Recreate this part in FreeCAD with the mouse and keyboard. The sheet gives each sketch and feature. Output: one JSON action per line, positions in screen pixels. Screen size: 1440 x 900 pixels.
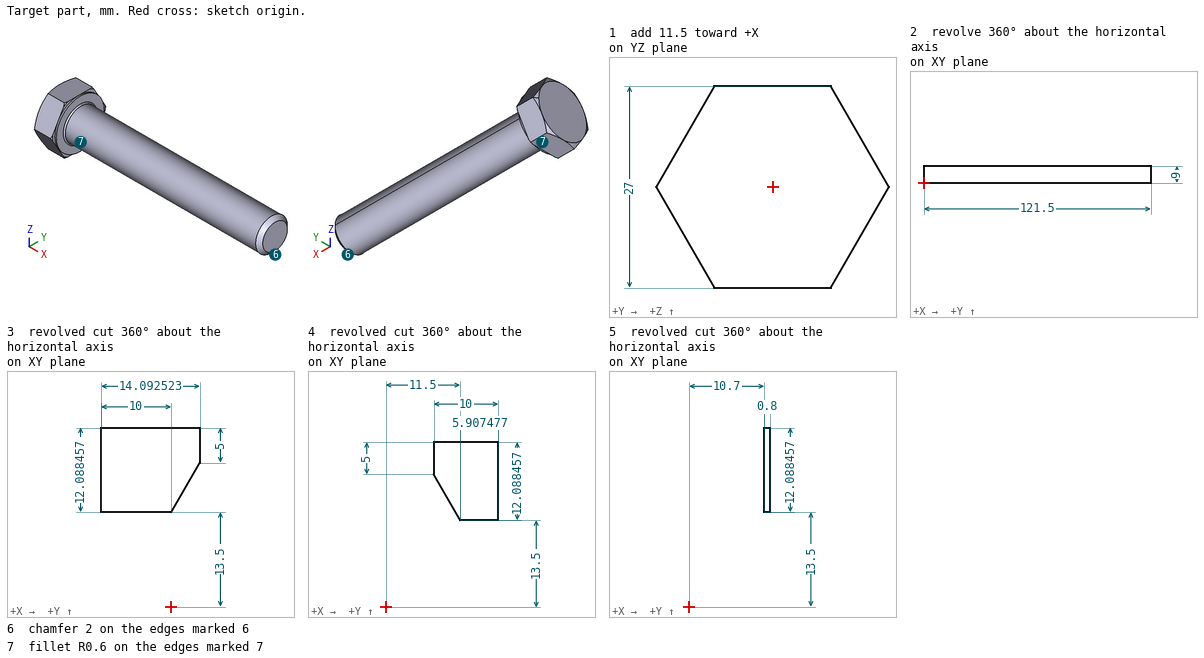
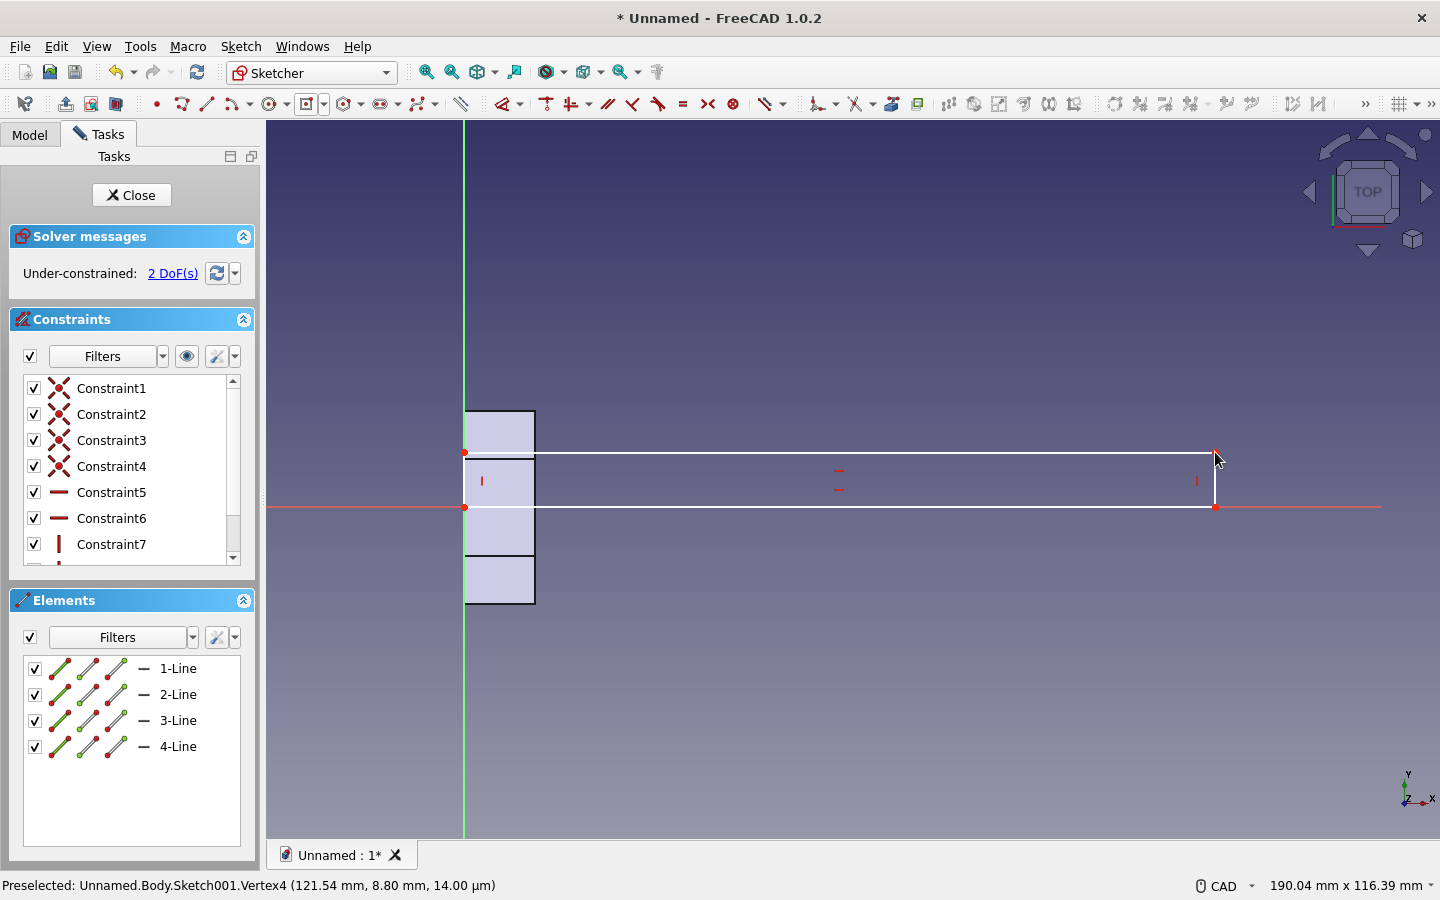
{"action": "left_click", "coordinate": [502, 104]}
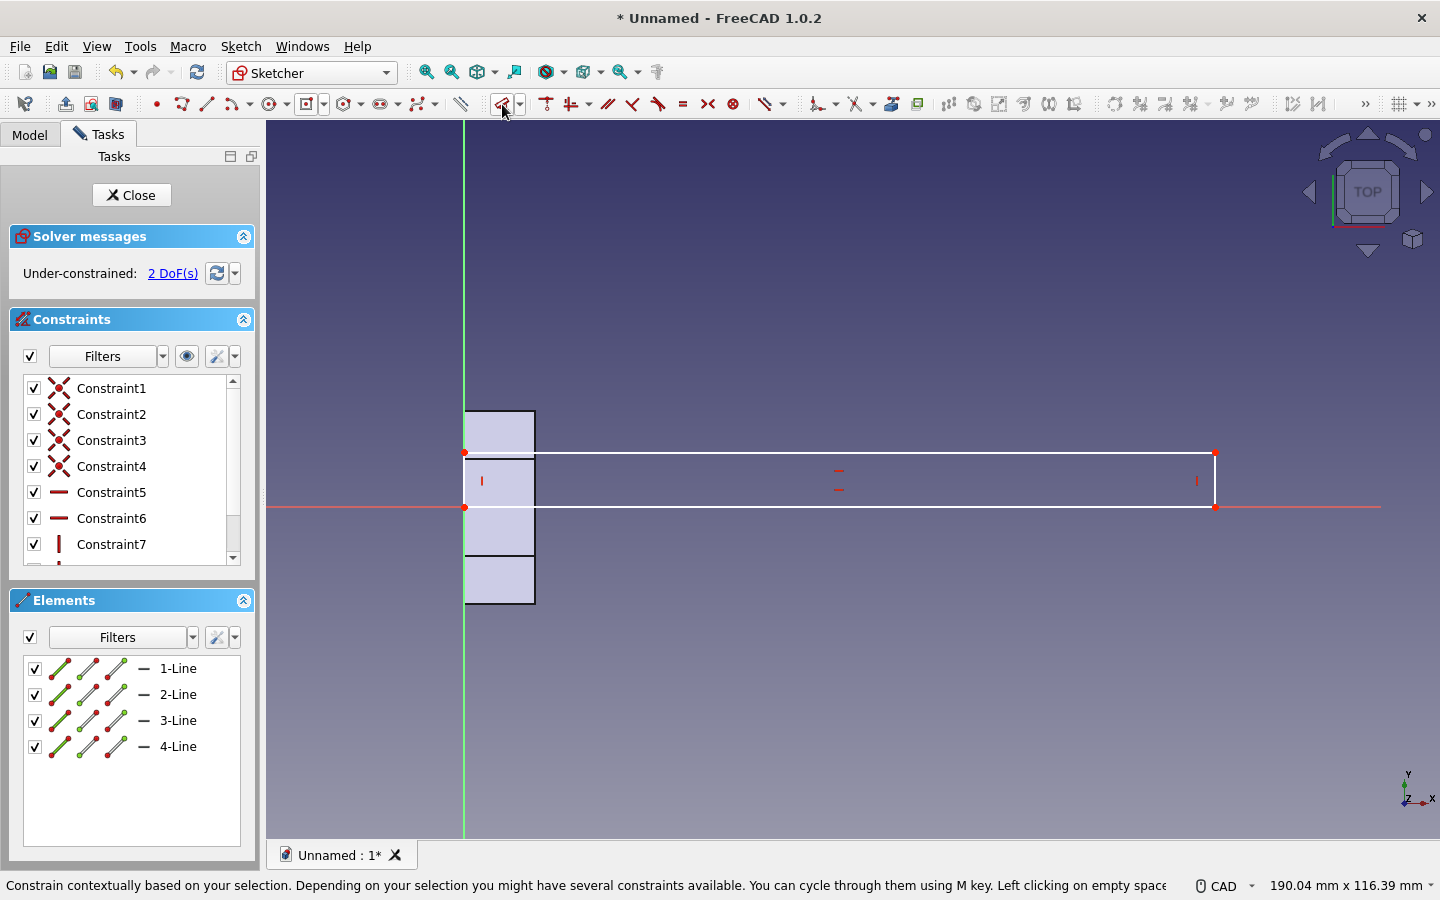
{"action": "left_click", "coordinate": [1215, 491]}
{"action": "left_click", "coordinate": [1249, 480]}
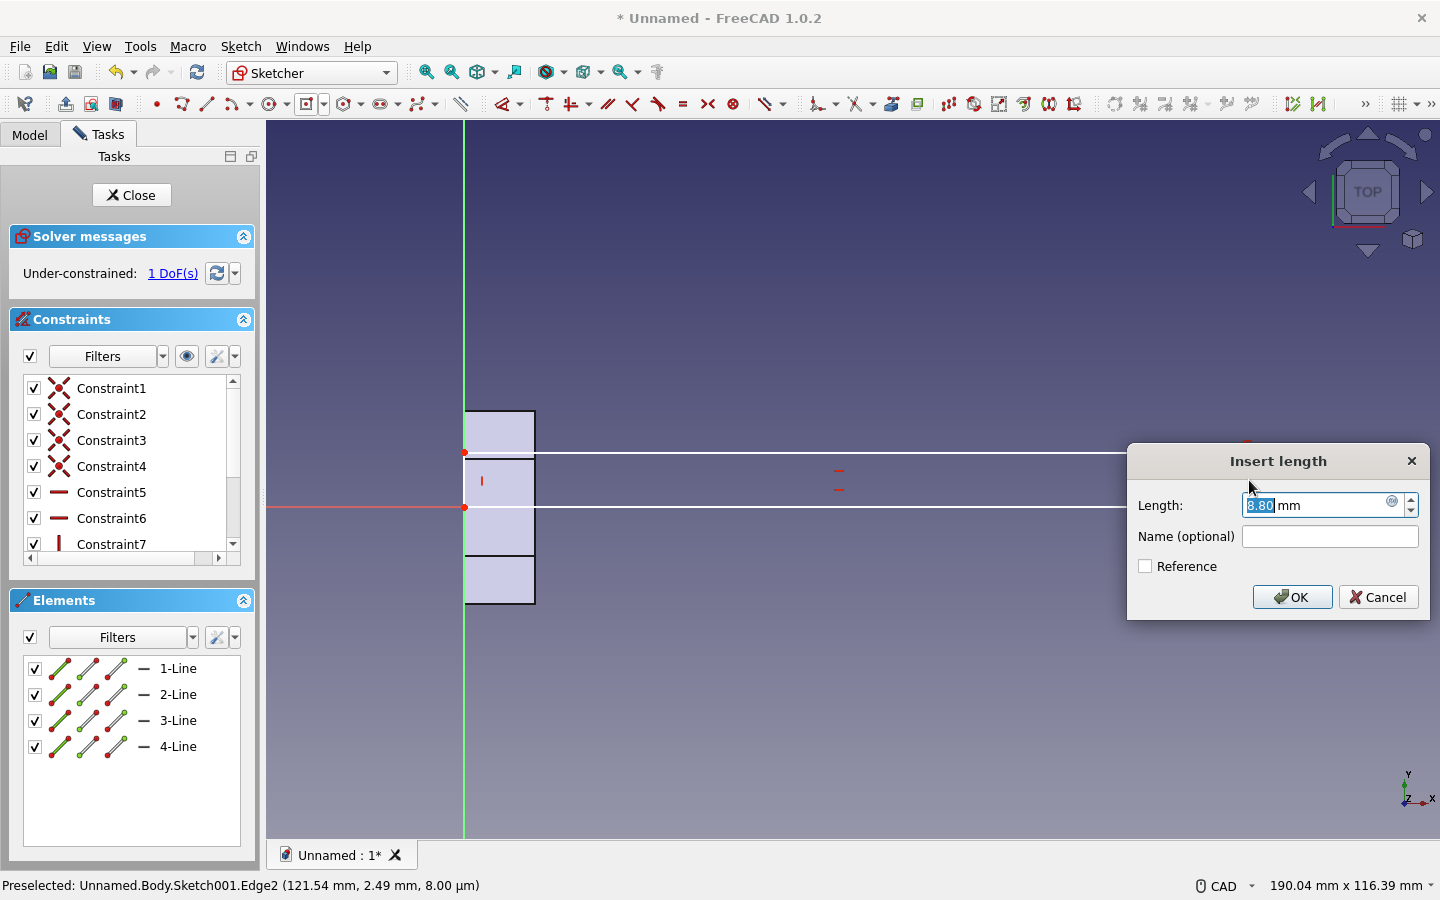
{"action": "type", "text": "9"}
{"action": "key", "text": "Return"}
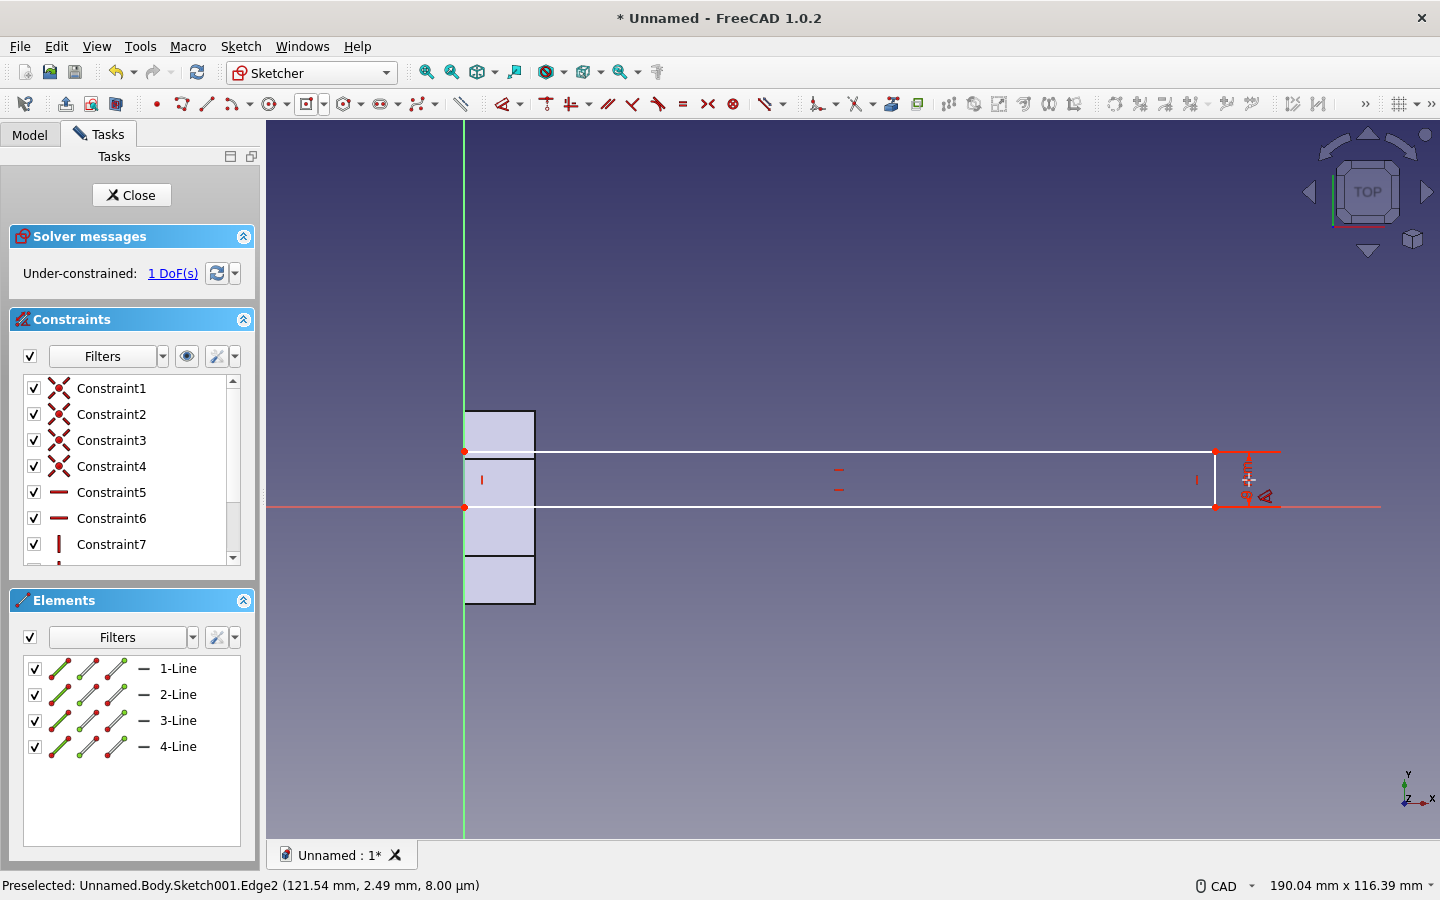
{"action": "left_click", "coordinate": [689, 507]}
{"action": "left_click", "coordinate": [840, 541]}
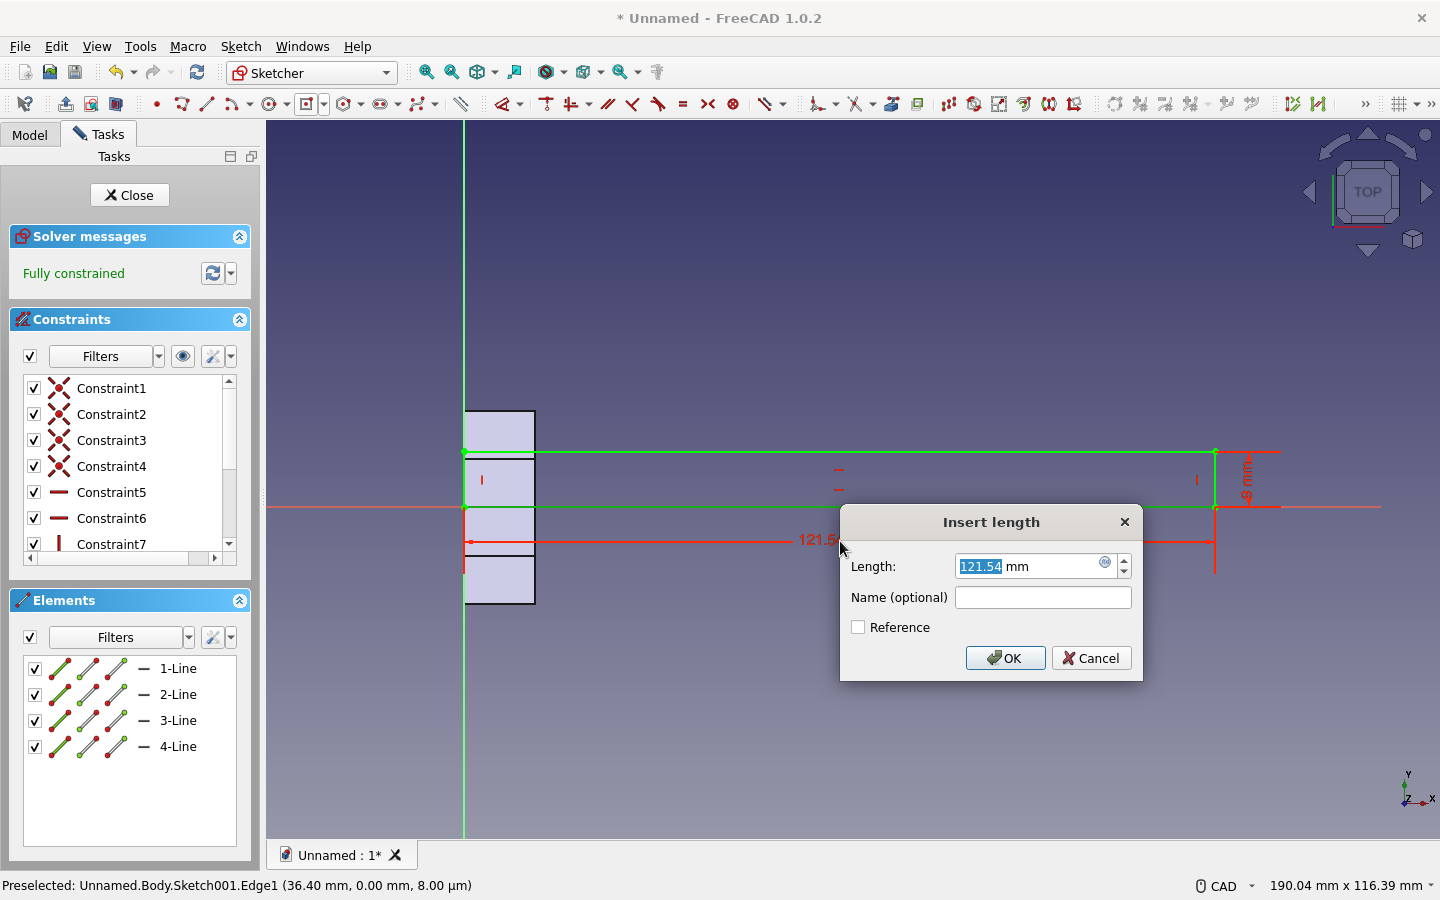
{"action": "type", "text": "121.5"}
{"action": "key", "text": "Return"}
{"action": "key", "text": "Escape"}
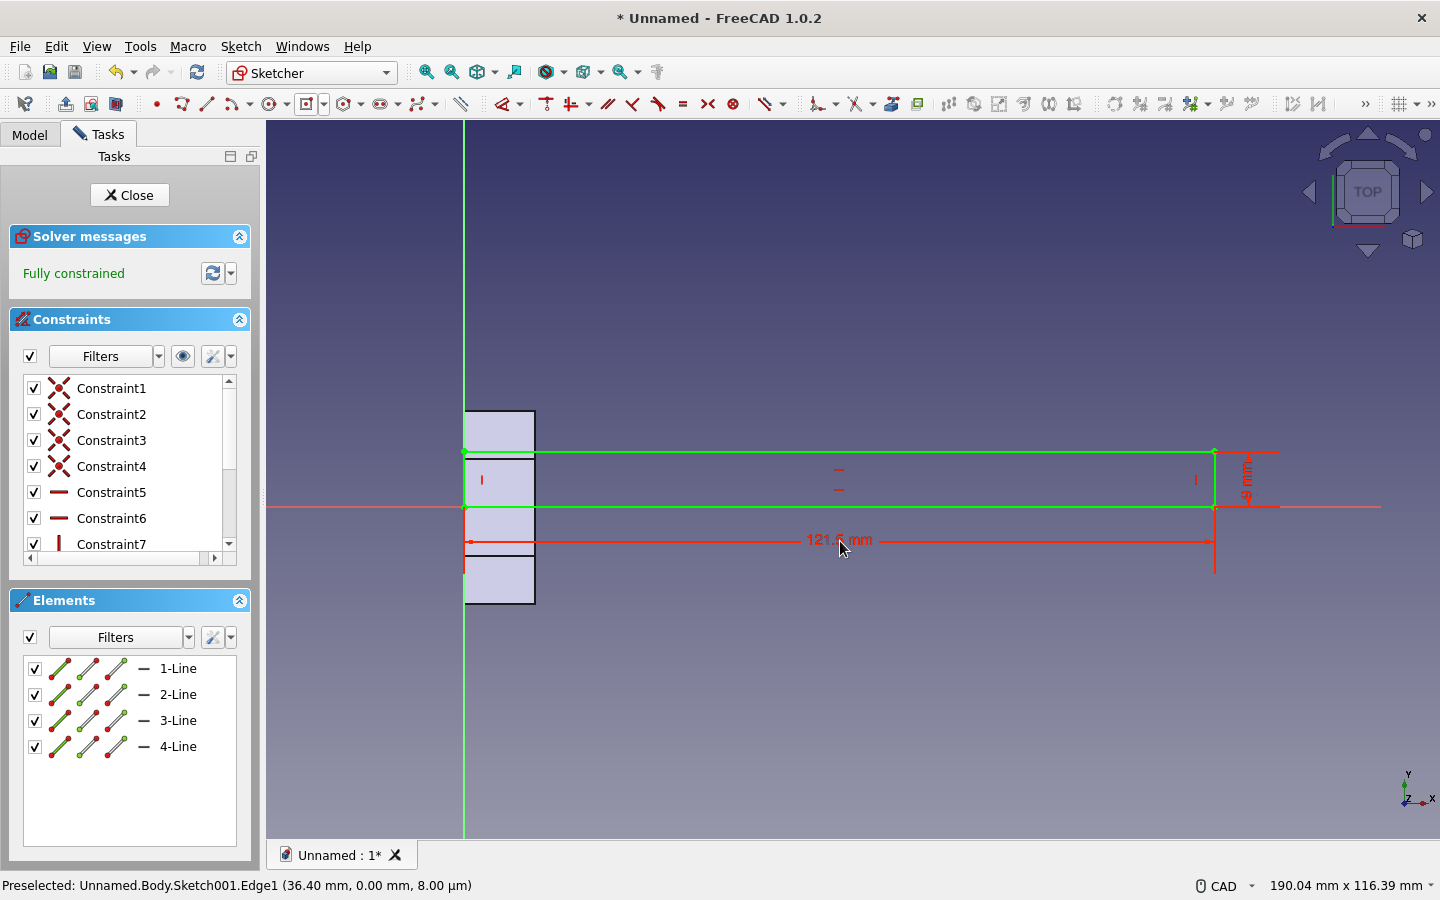
{"action": "left_click", "coordinate": [130, 195]}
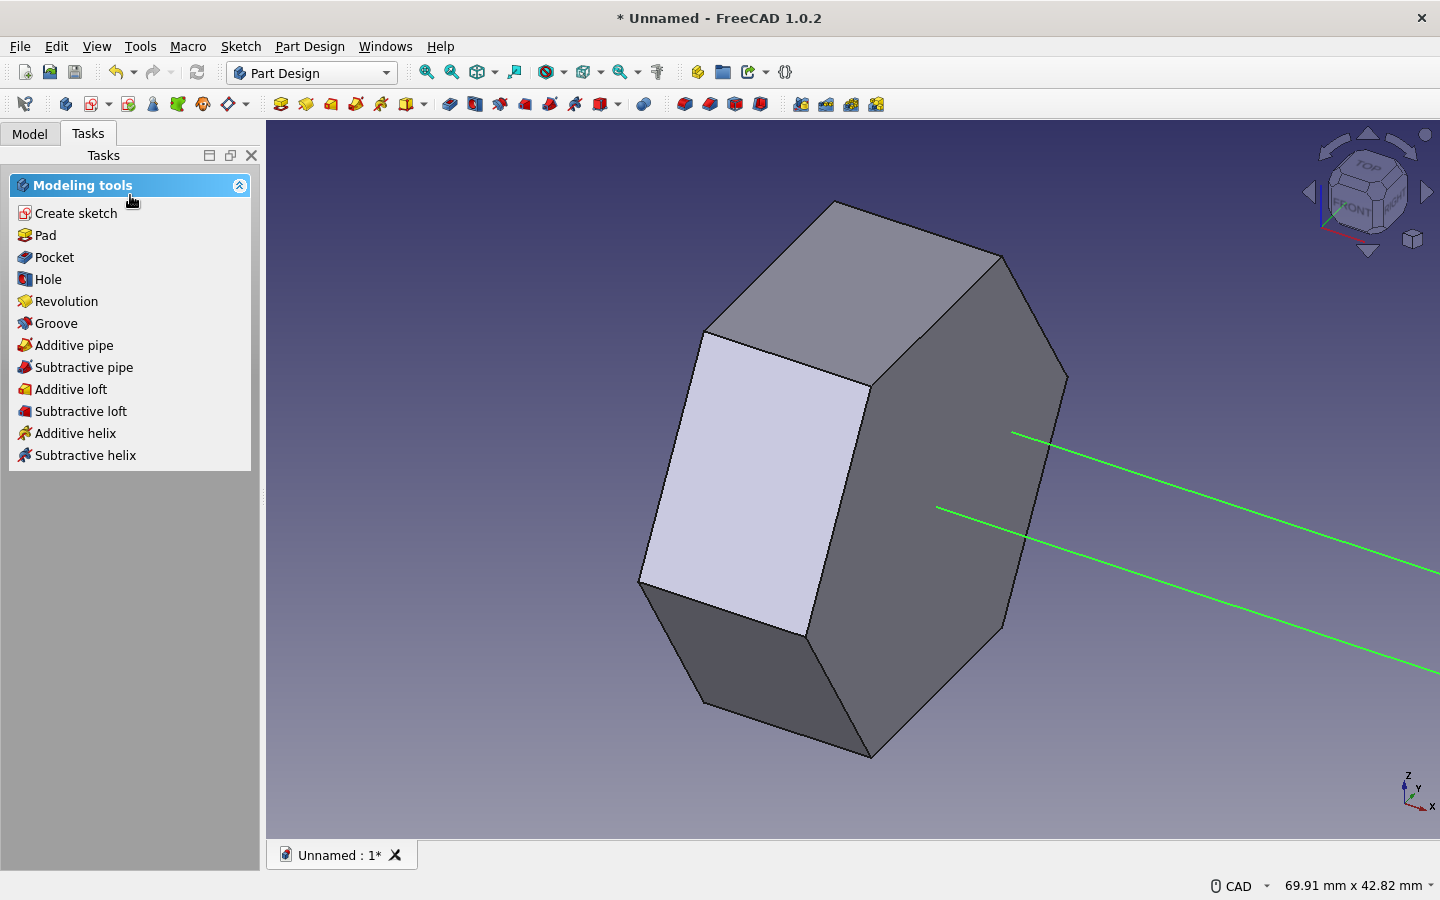
{"action": "left_click", "coordinate": [306, 104]}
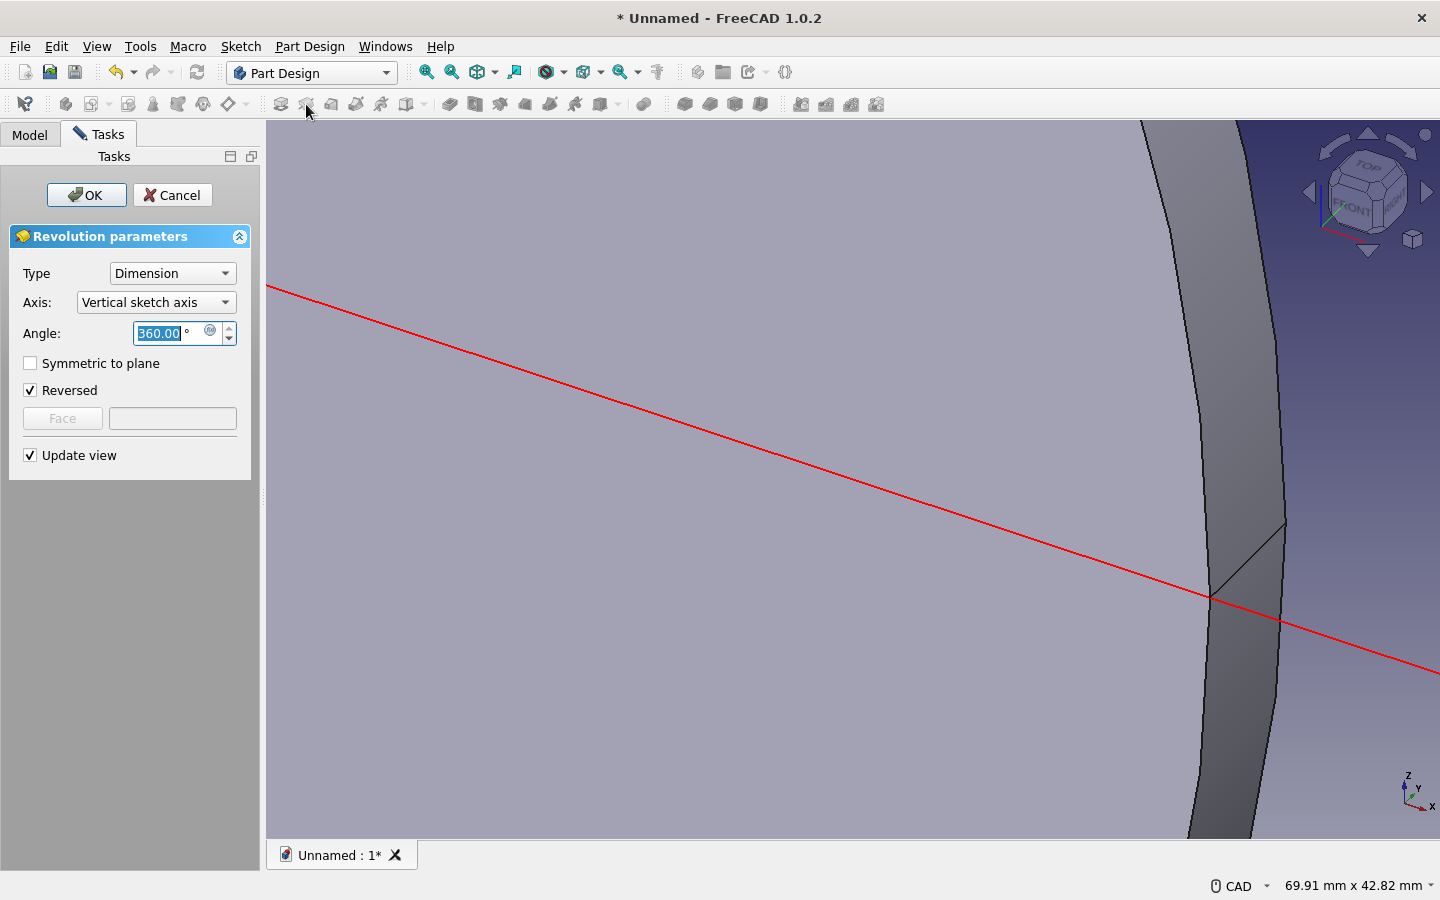
{"action": "left_click", "coordinate": [157, 302]}